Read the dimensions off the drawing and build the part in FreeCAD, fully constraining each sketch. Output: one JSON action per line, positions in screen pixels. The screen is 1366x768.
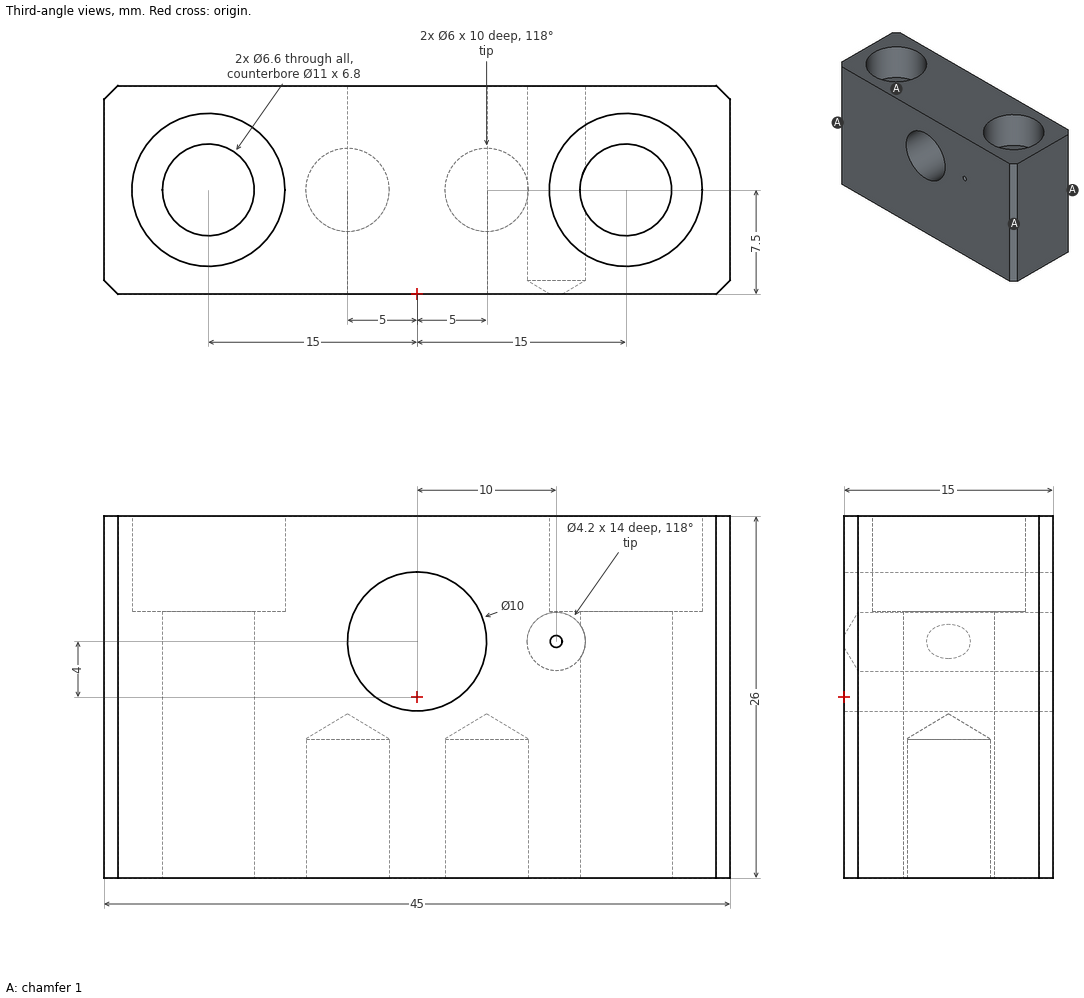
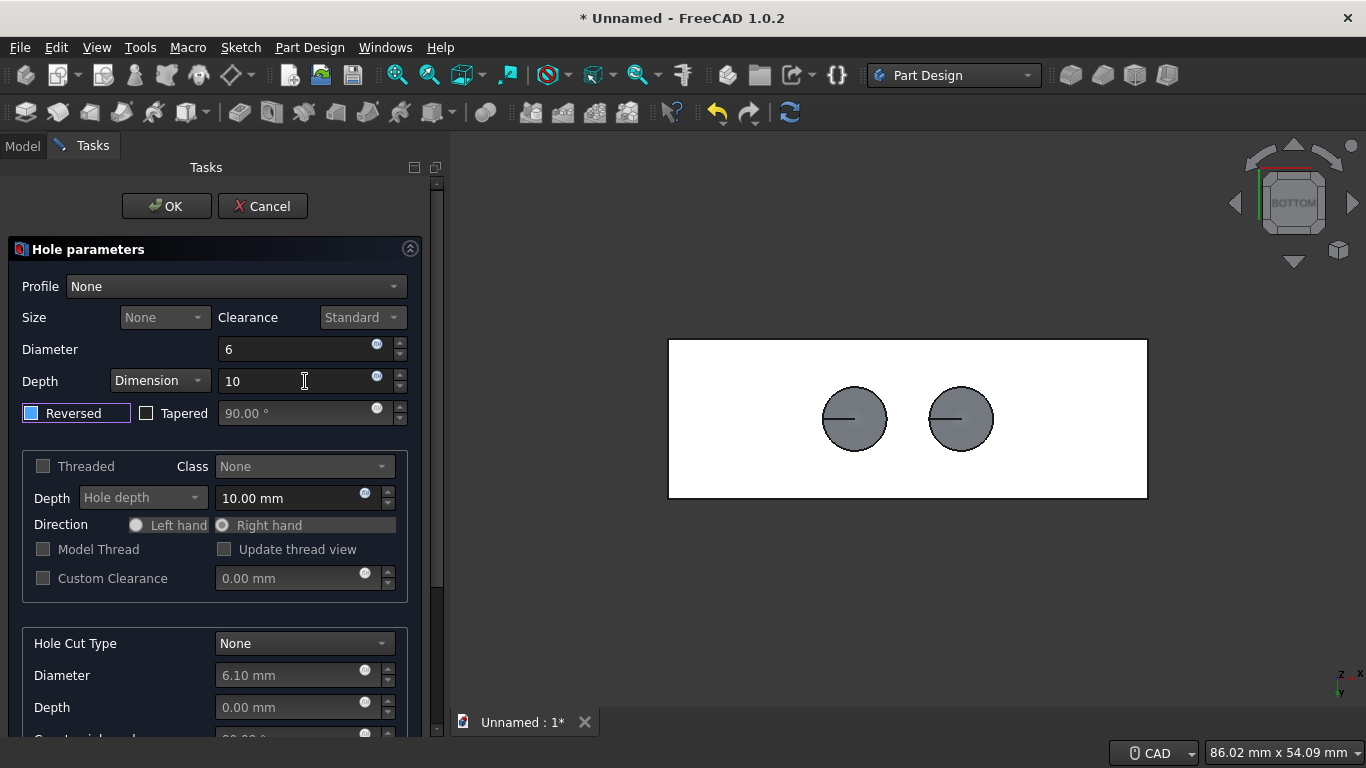
{"action": "left_click", "coordinate": [167, 206]}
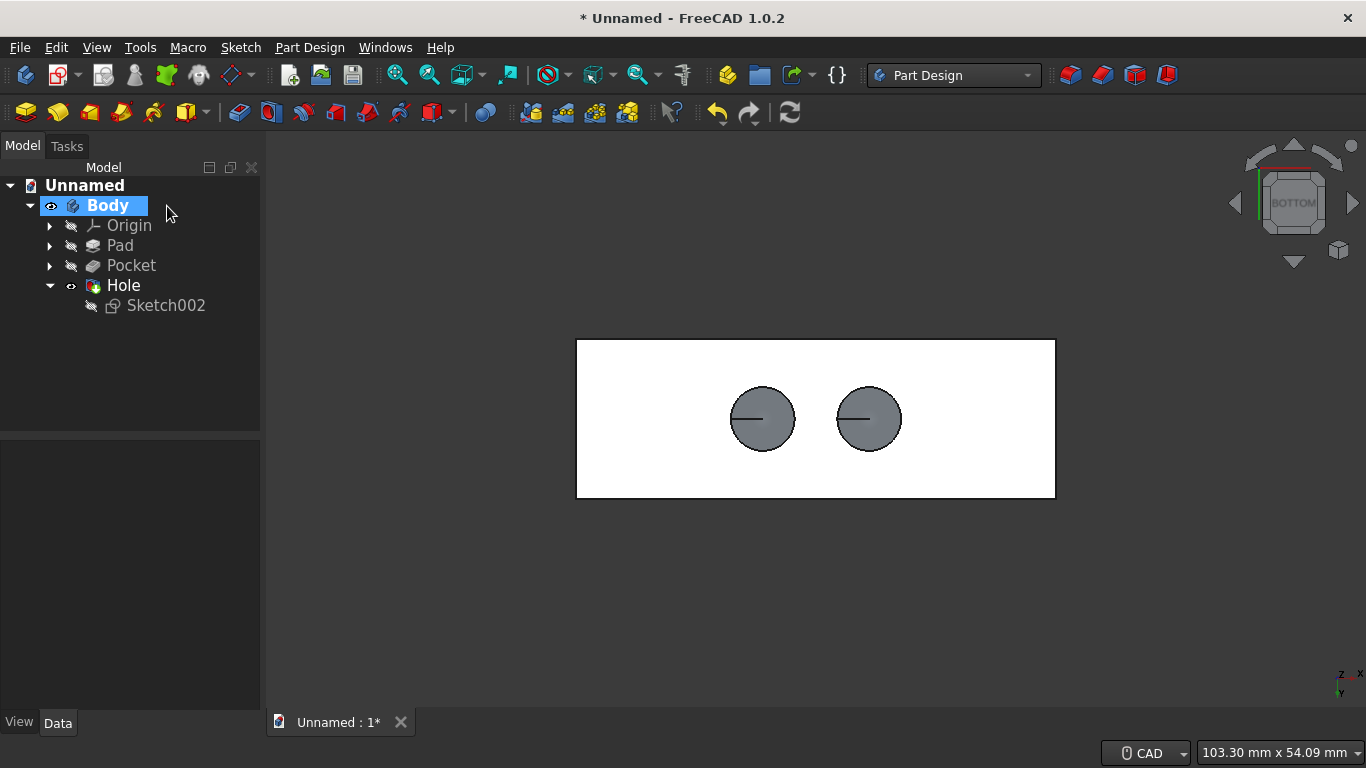
{"action": "left_click", "coordinate": [398, 76]}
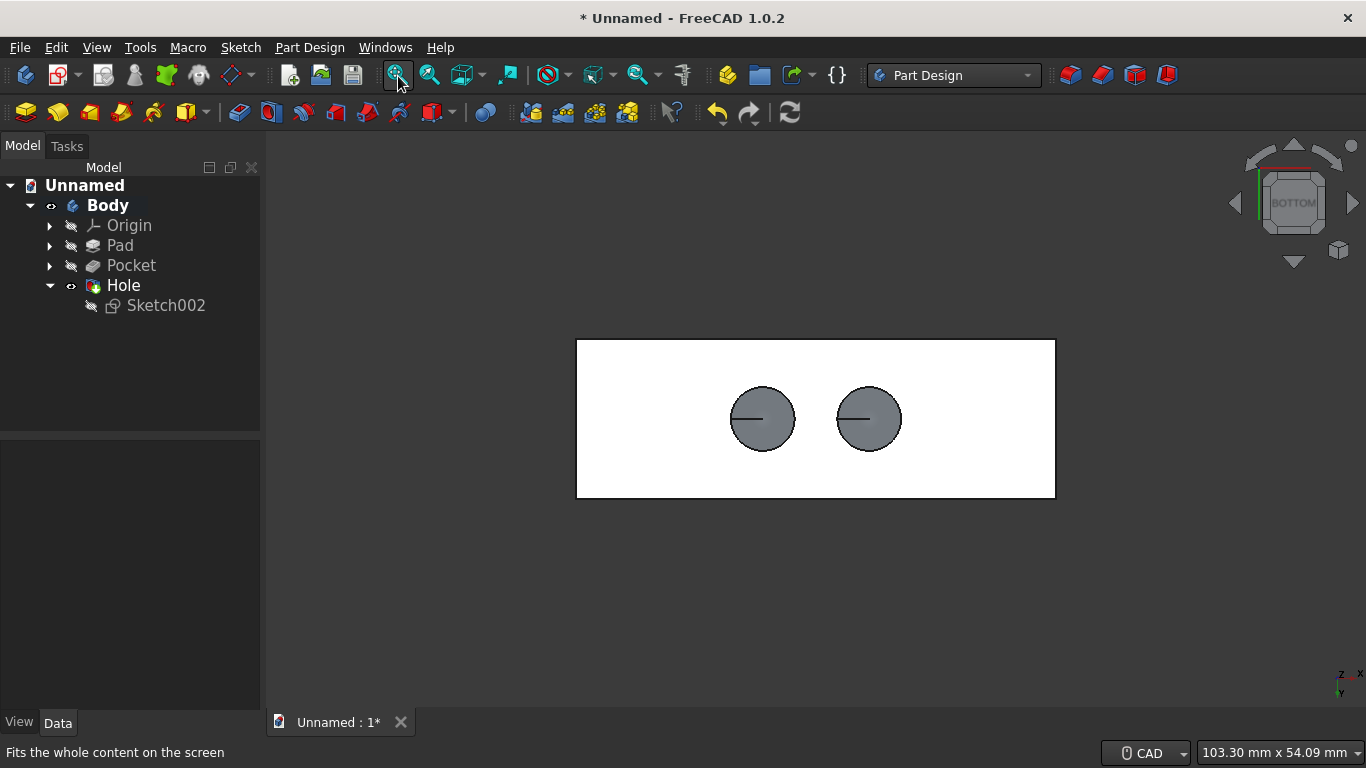
{"action": "key", "text": "0"}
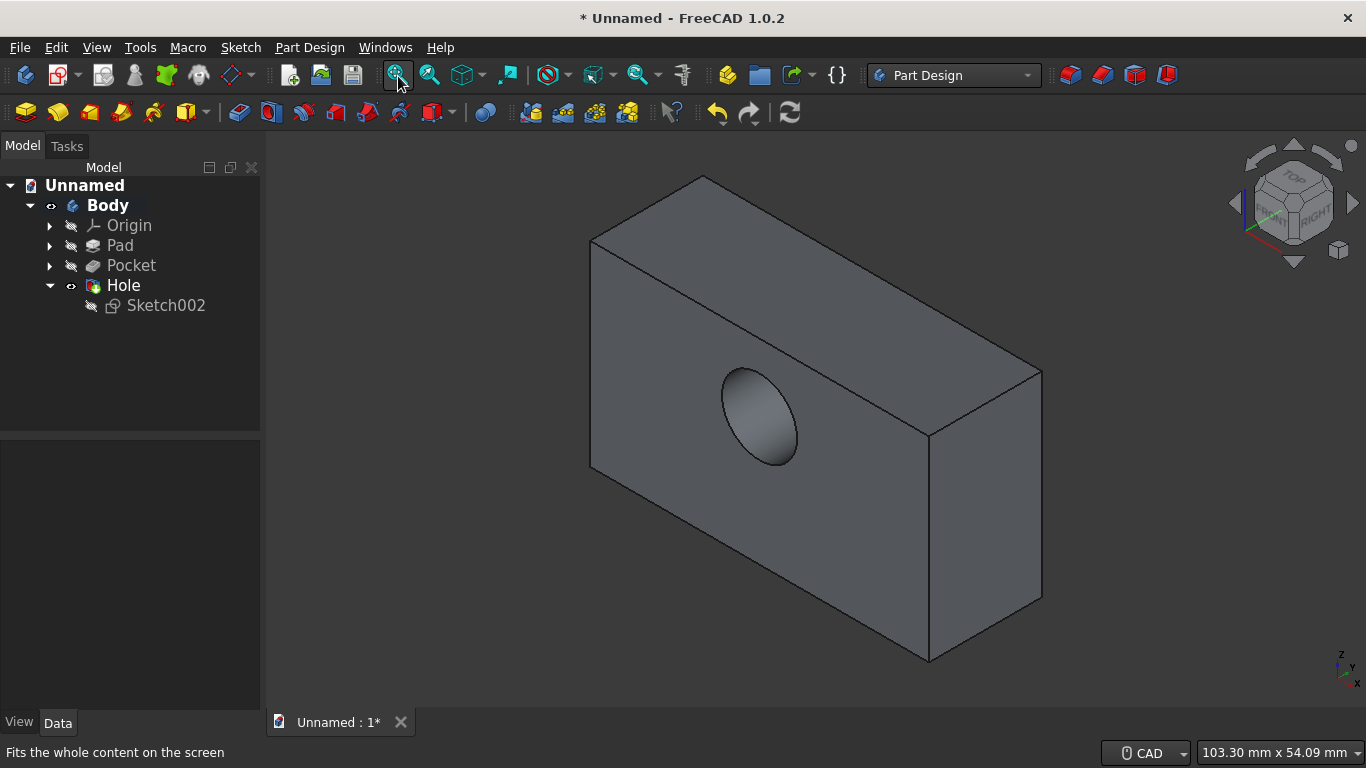
{"action": "left_click", "coordinate": [929, 548]}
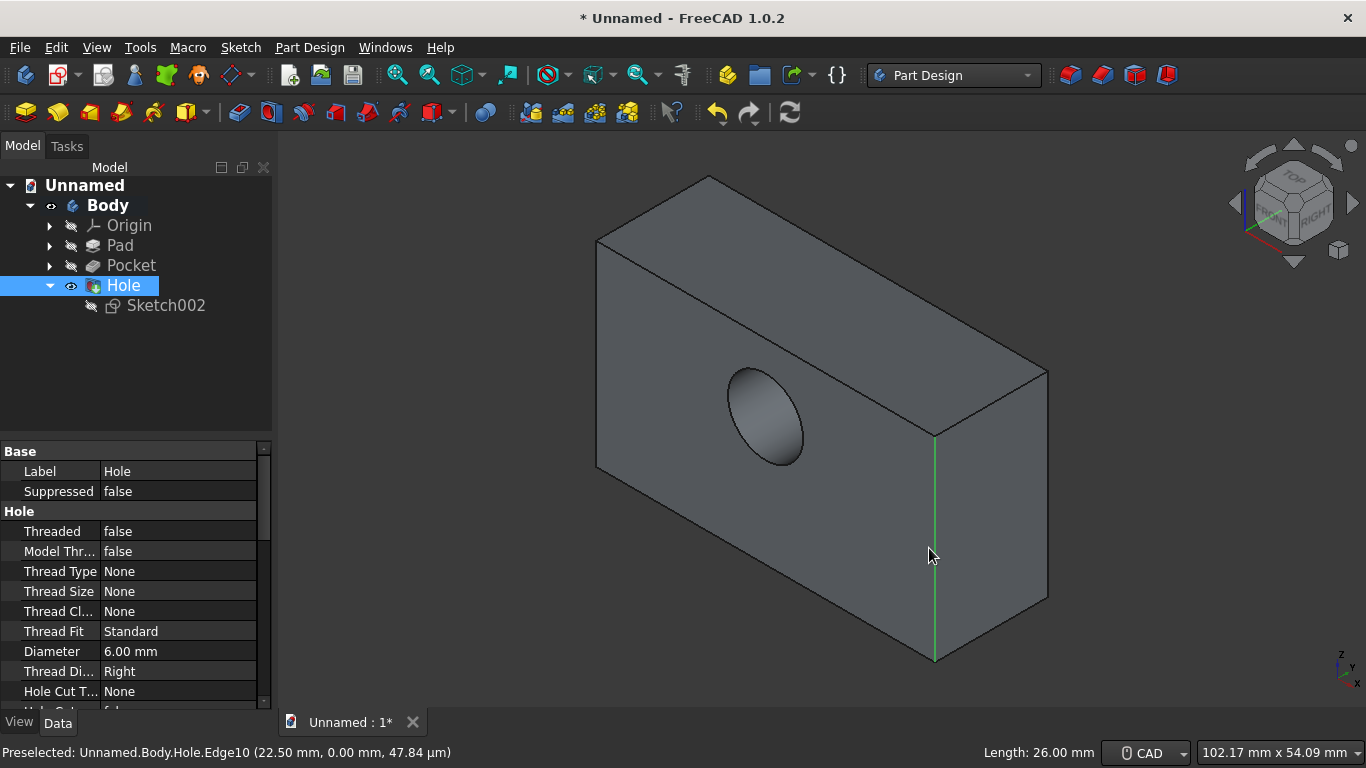
{"action": "key", "text": "2"}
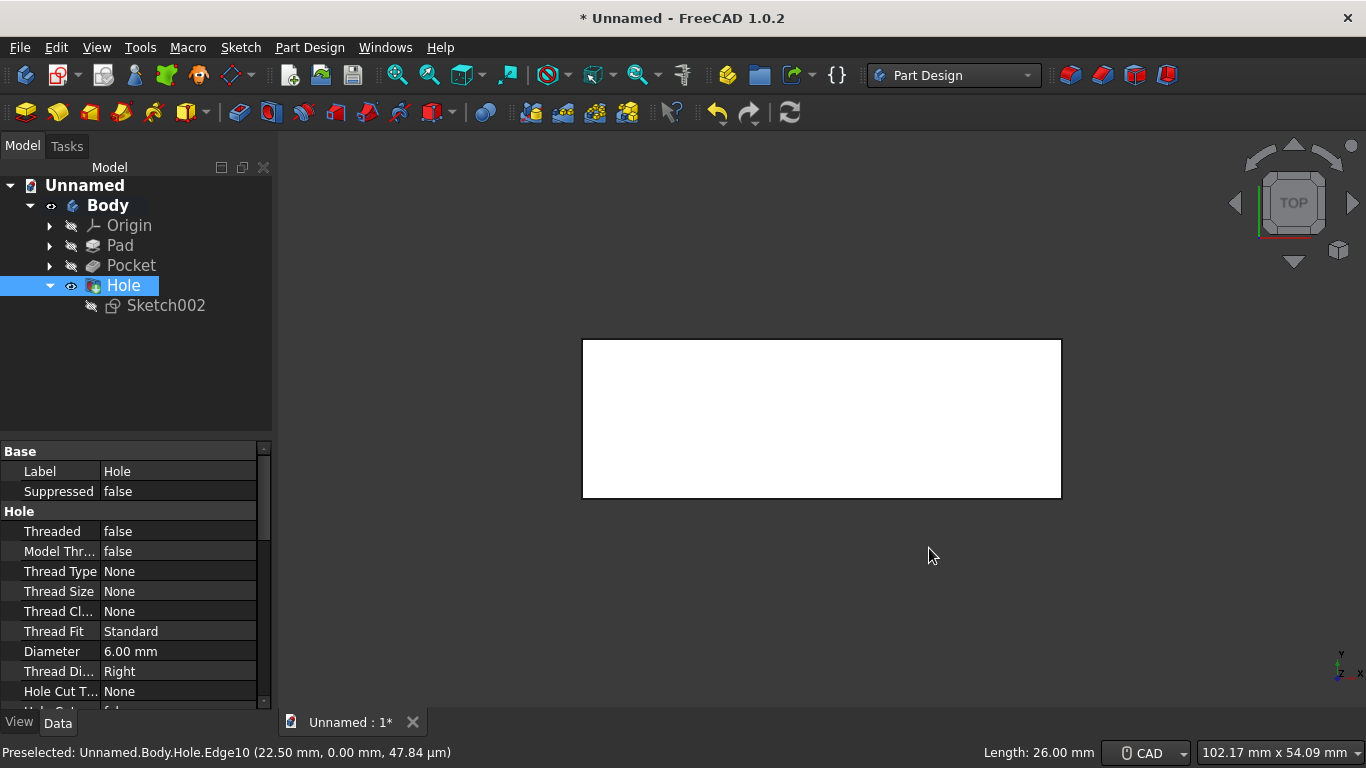
{"action": "left_click", "coordinate": [398, 76]}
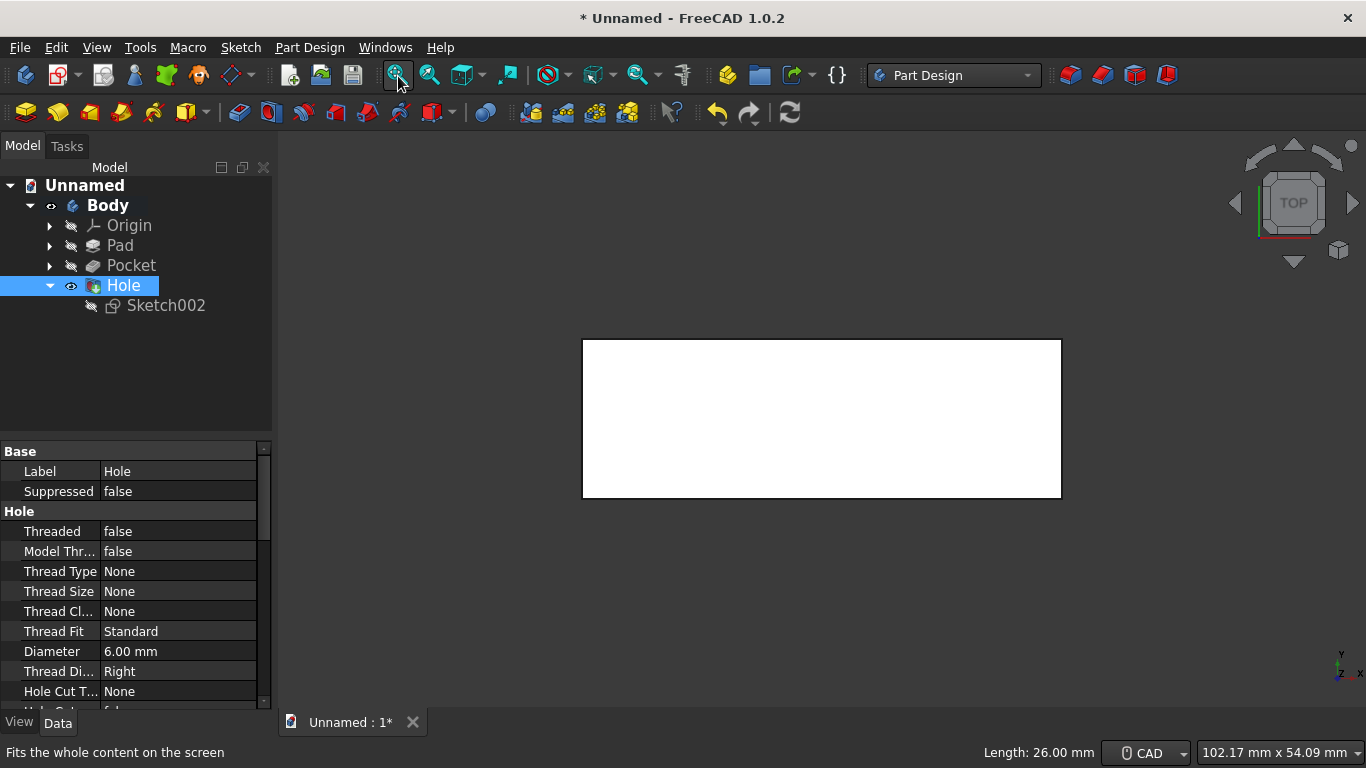
{"action": "key", "text": "1"}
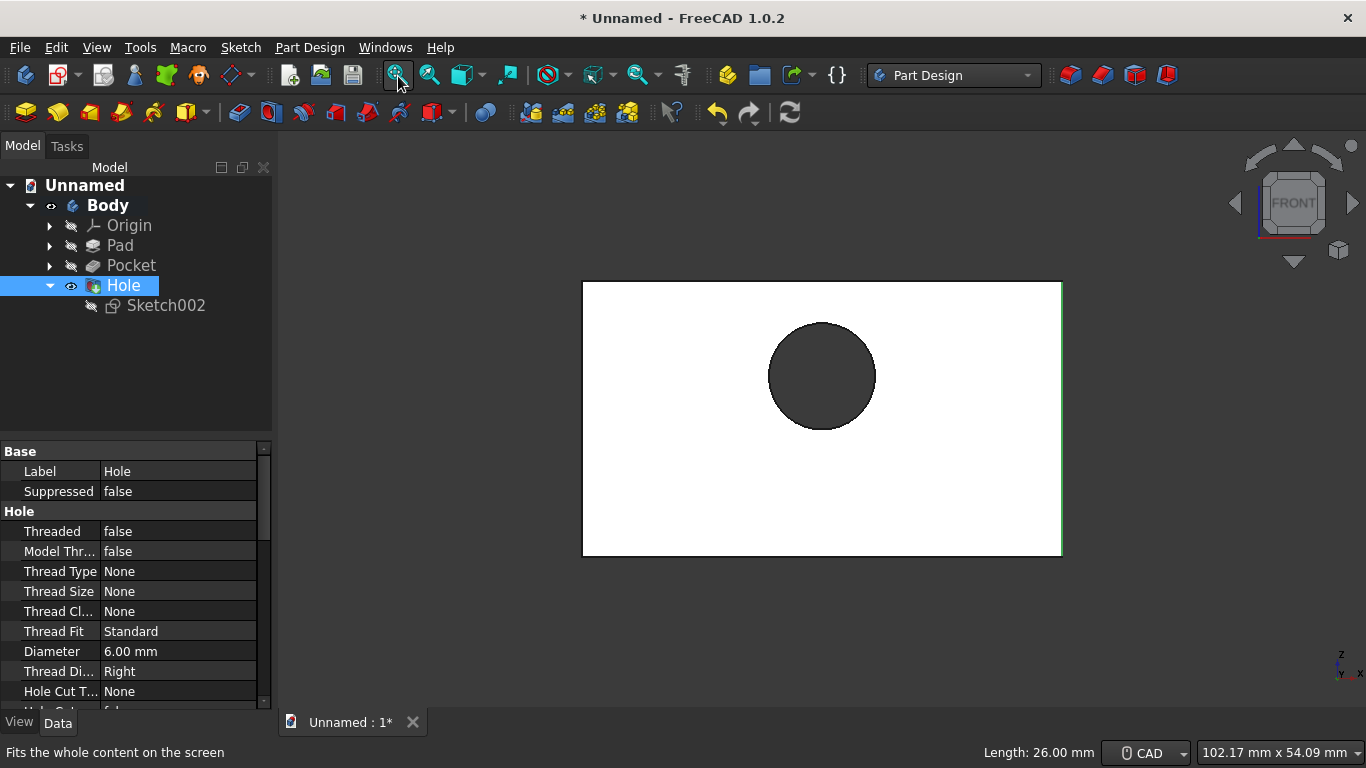
{"action": "key", "text": "3"}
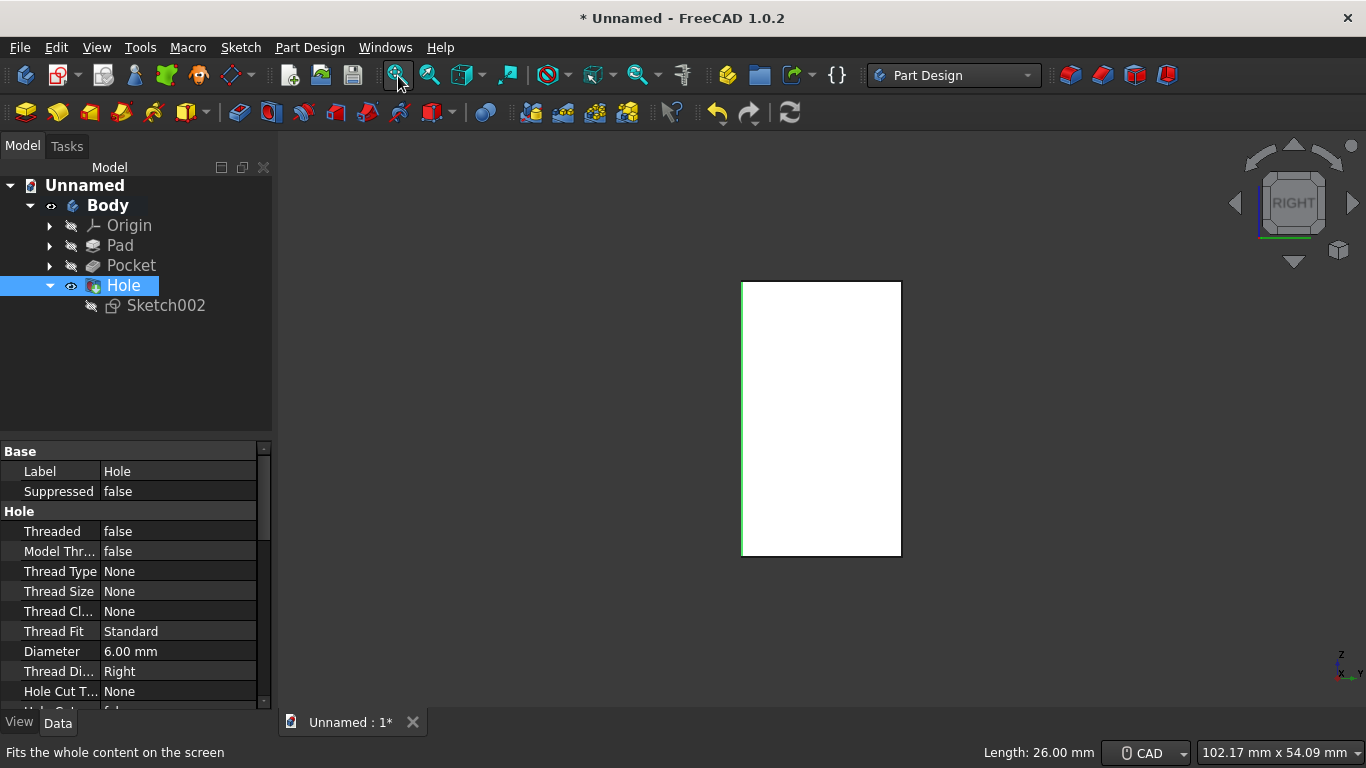
{"action": "left_click", "coordinate": [902, 418], "text": "ctrl"}